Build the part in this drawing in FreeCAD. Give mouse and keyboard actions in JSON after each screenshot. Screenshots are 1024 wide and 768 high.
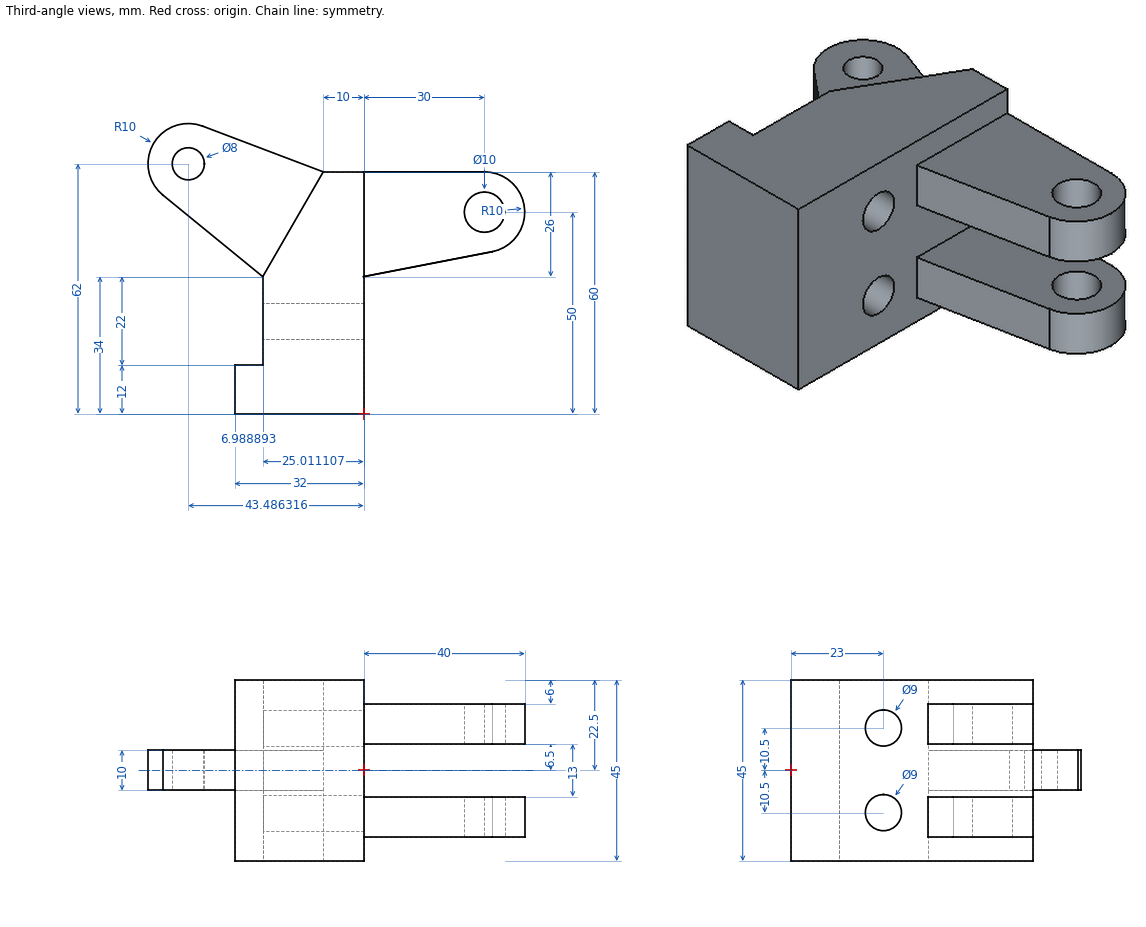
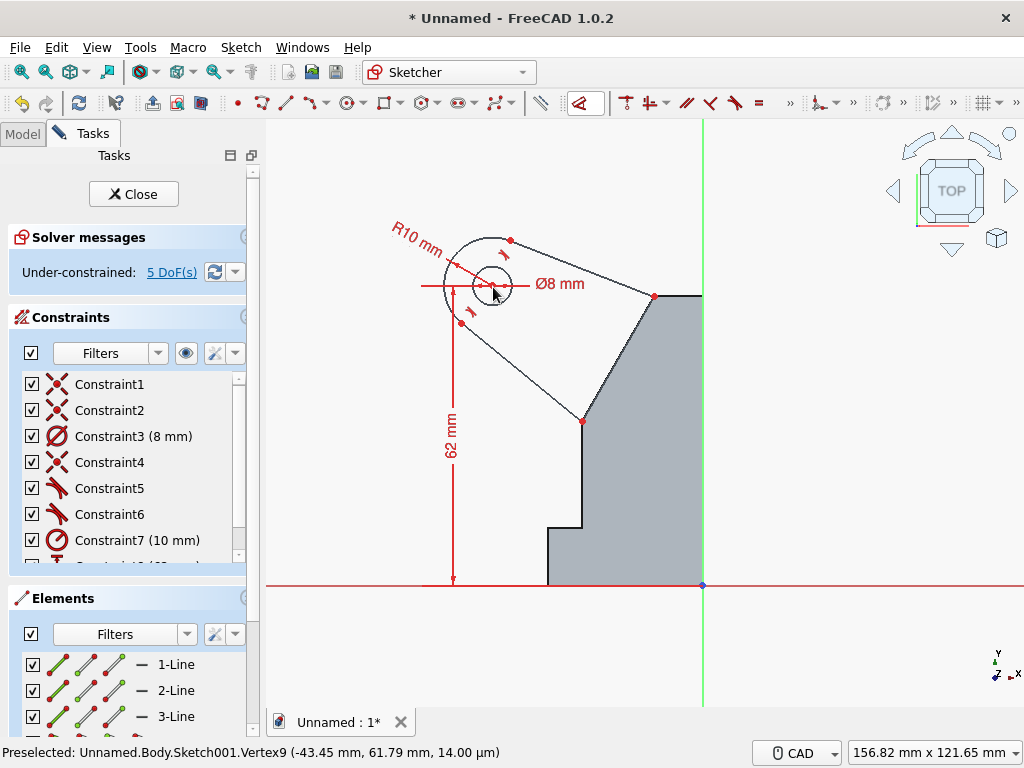
{"action": "left_click", "coordinate": [582, 422]}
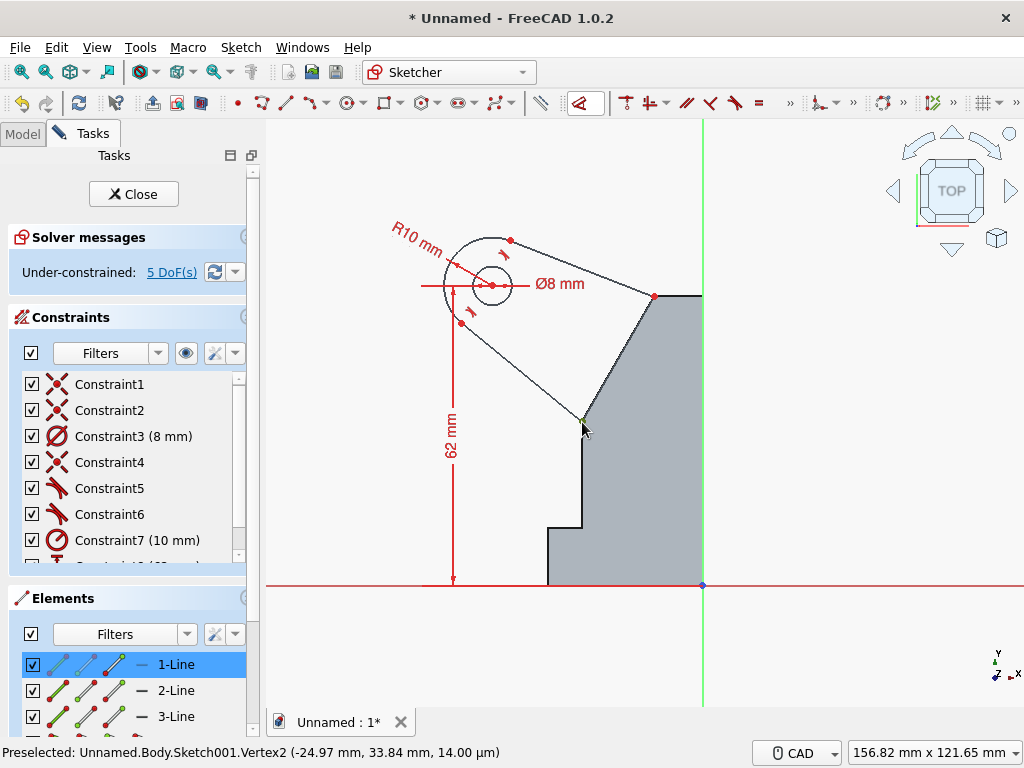
{"action": "key", "text": "i"}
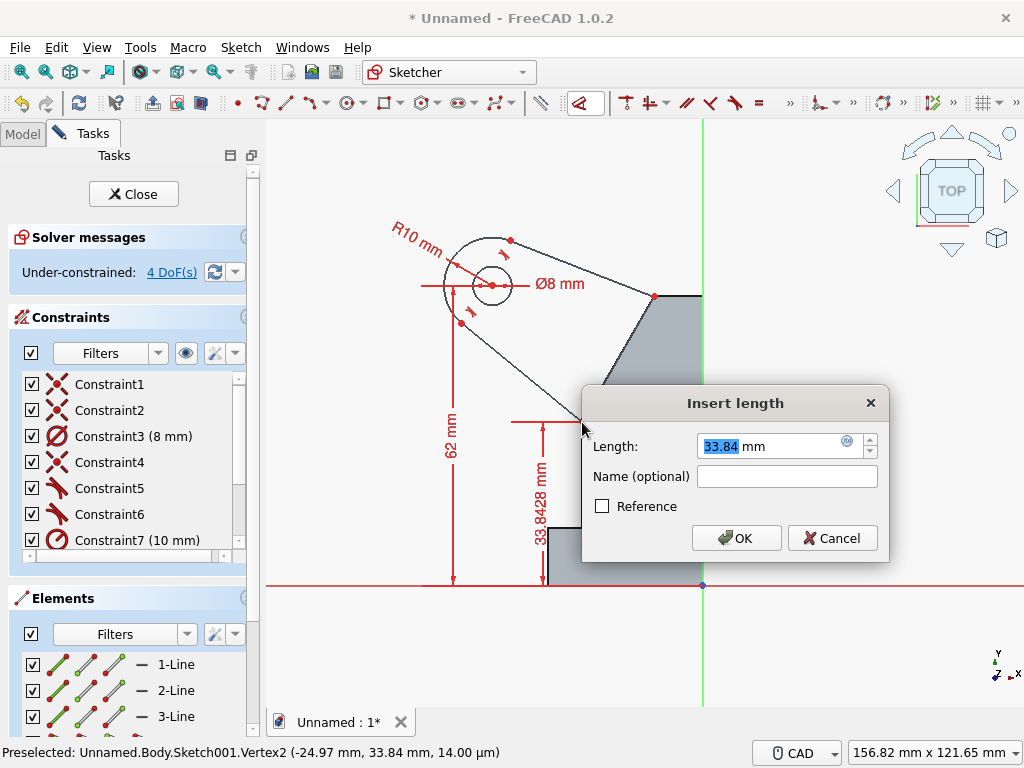
{"action": "type", "text": "34"}
{"action": "key", "text": "Return"}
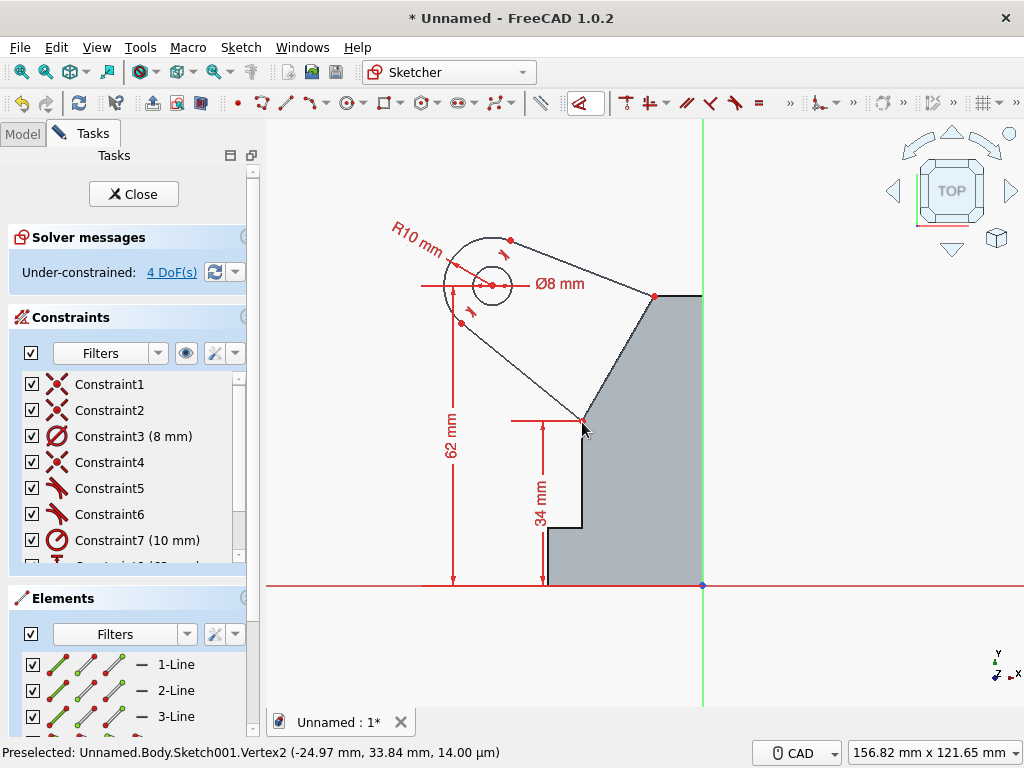
{"action": "left_click", "coordinate": [654, 297]}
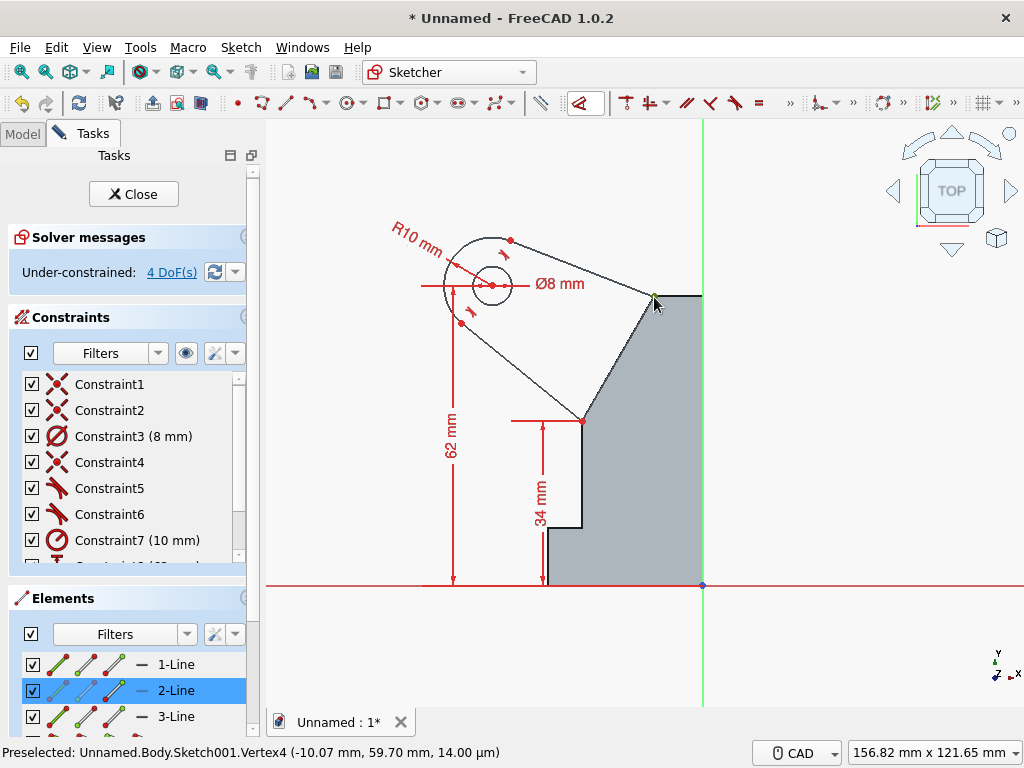
{"action": "key", "text": "l"}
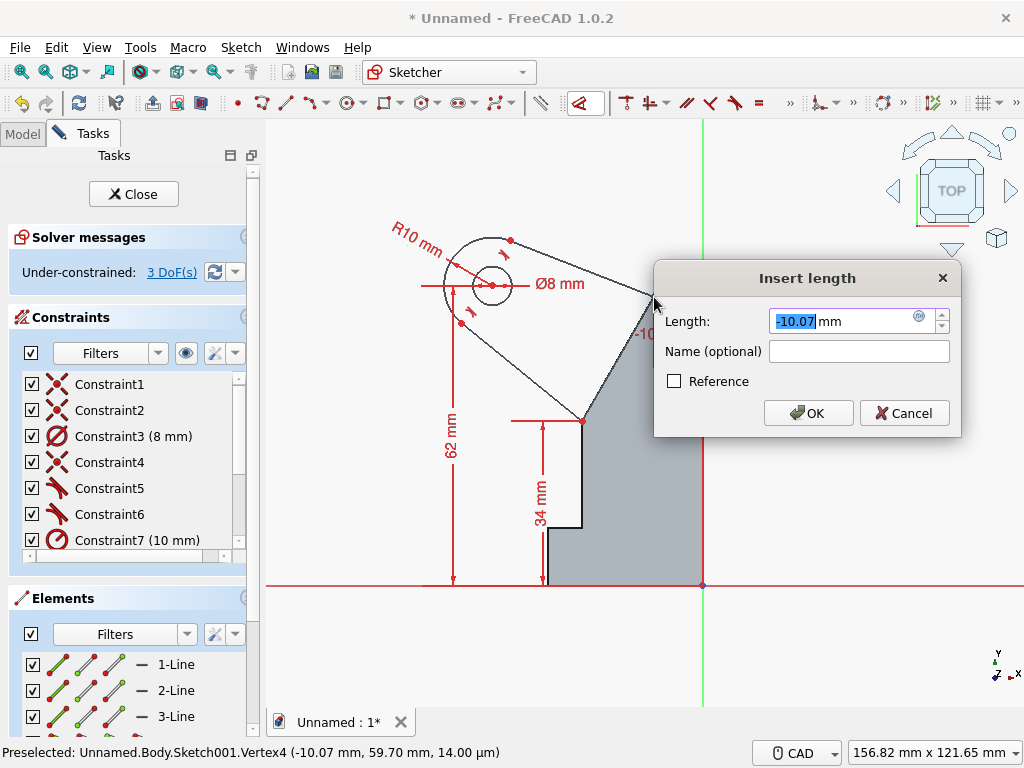
{"action": "type", "text": "-10"}
{"action": "key", "text": "Return"}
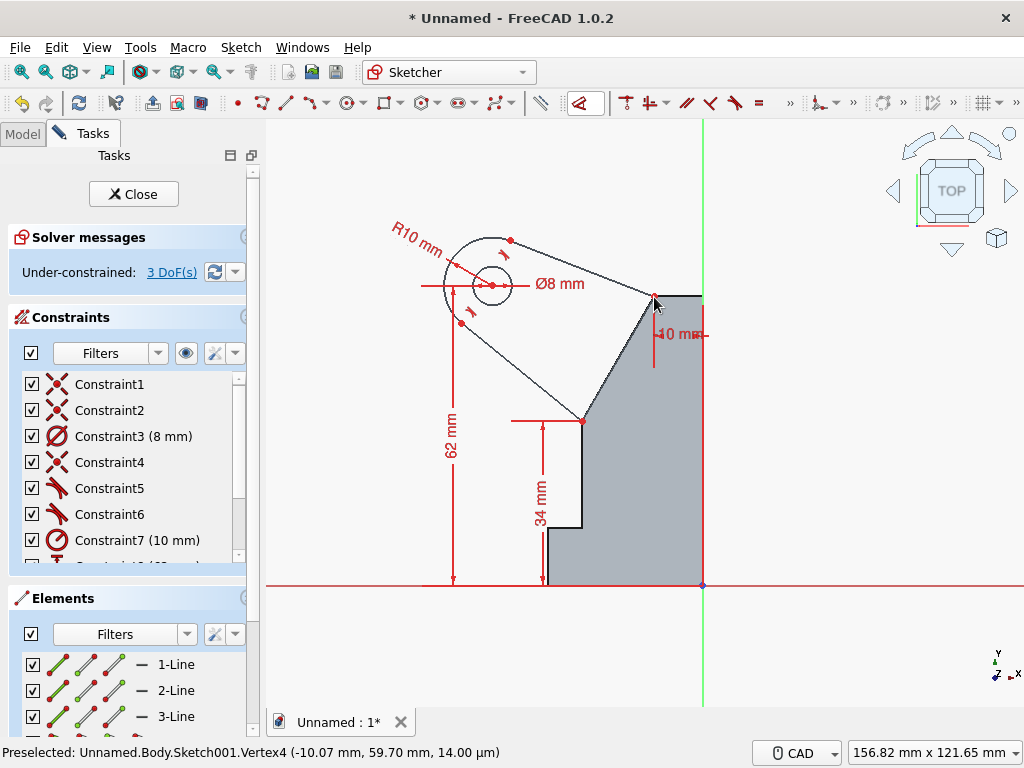
{"action": "left_click", "coordinate": [654, 297]}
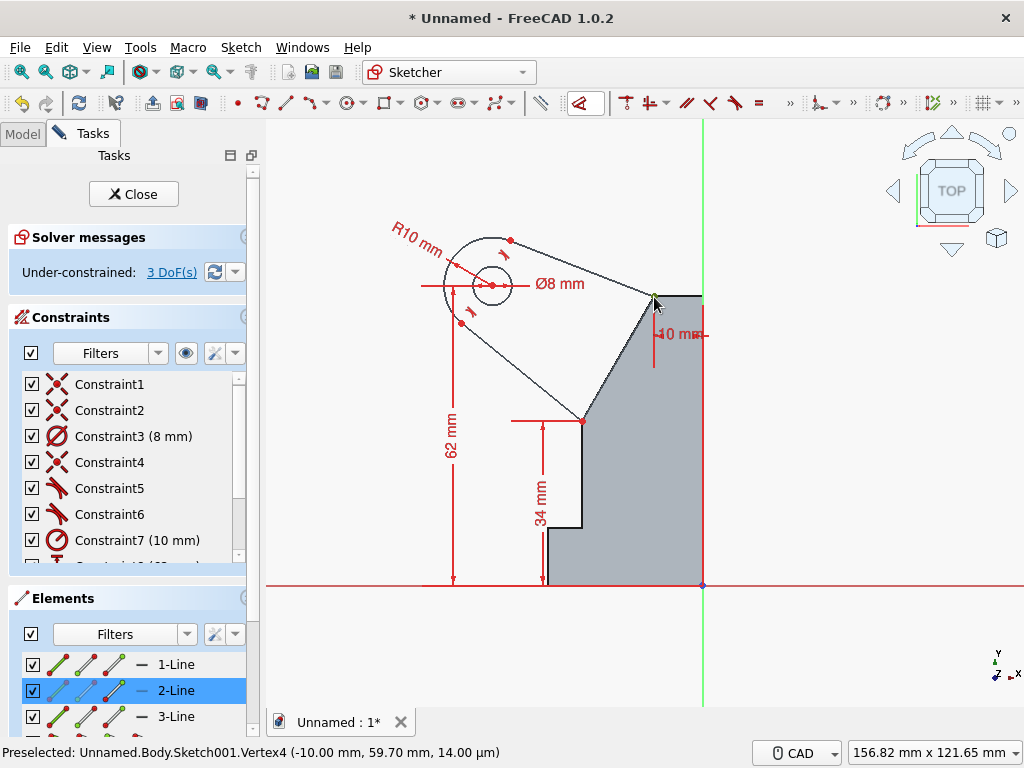
{"action": "key", "text": "i"}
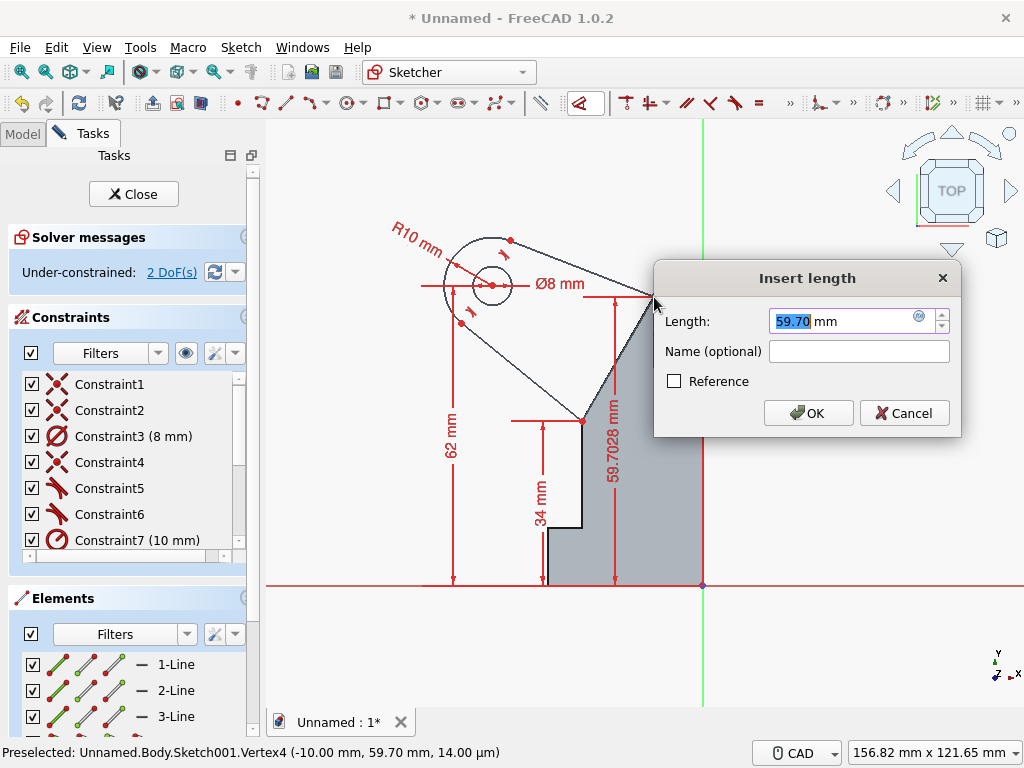
{"action": "type", "text": "60"}
{"action": "key", "text": "Return"}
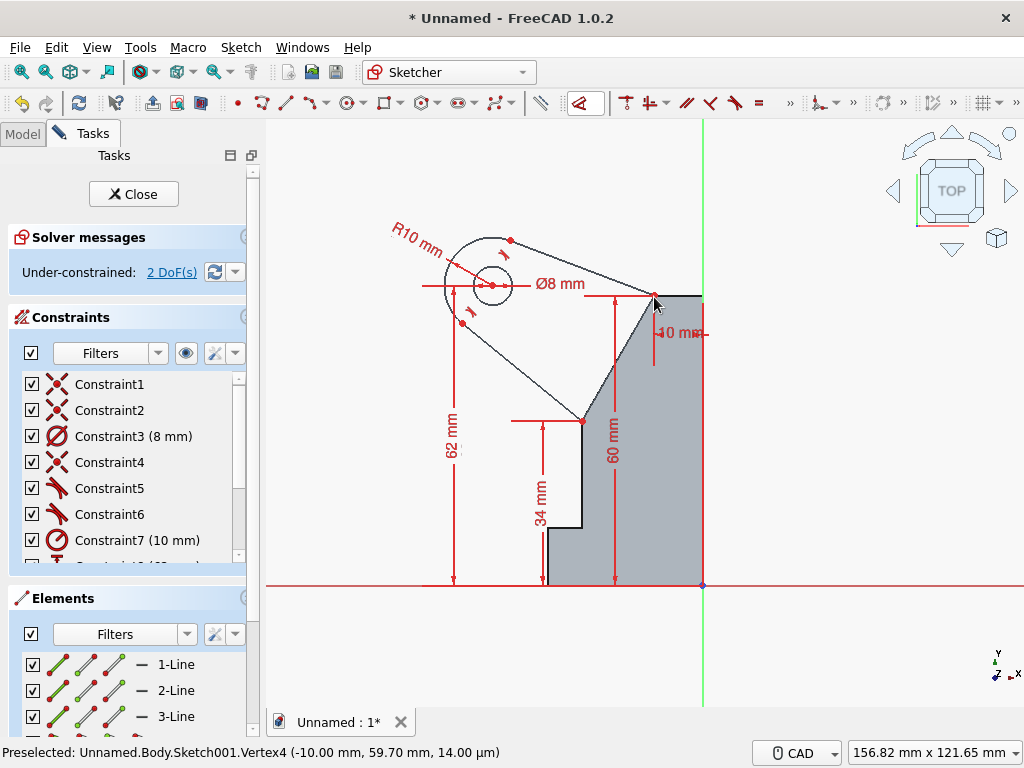
{"action": "left_click", "coordinate": [493, 286]}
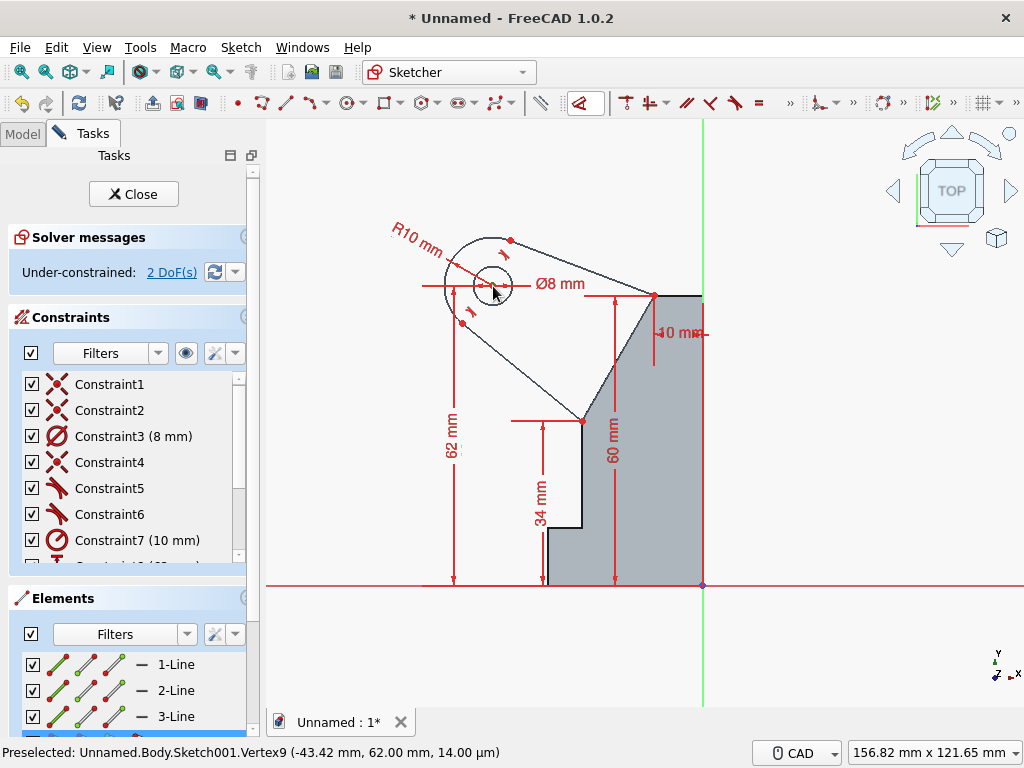
{"action": "key", "text": "l"}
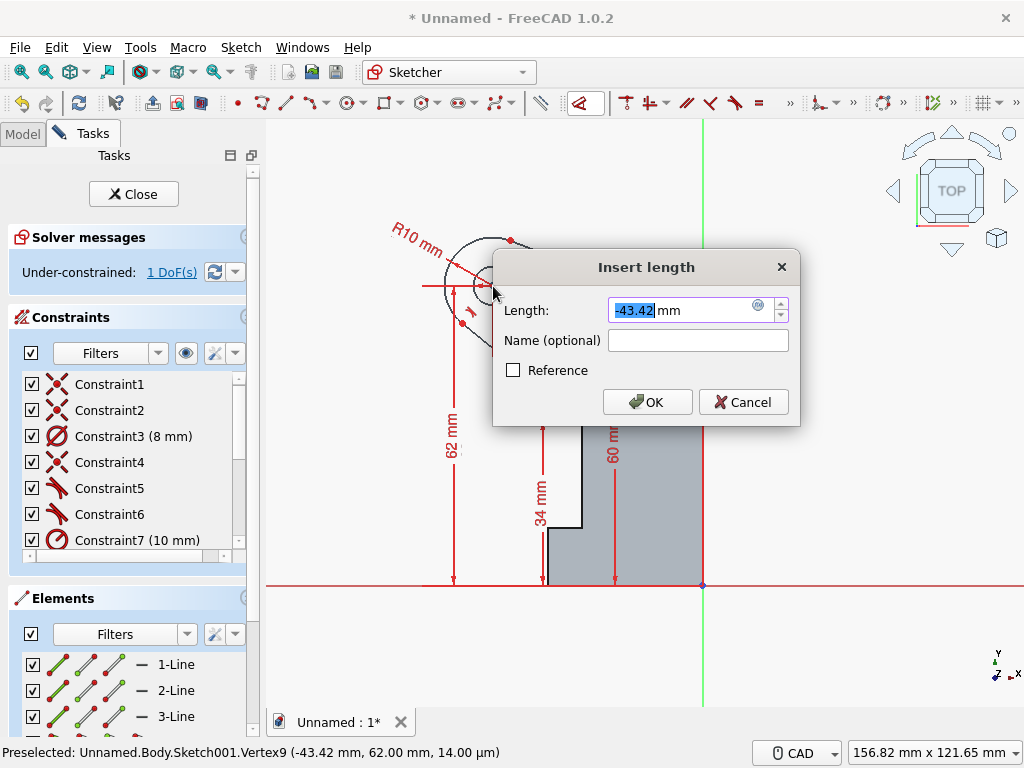
{"action": "type", "text": "-43.486316"}
{"action": "key", "text": "Return"}